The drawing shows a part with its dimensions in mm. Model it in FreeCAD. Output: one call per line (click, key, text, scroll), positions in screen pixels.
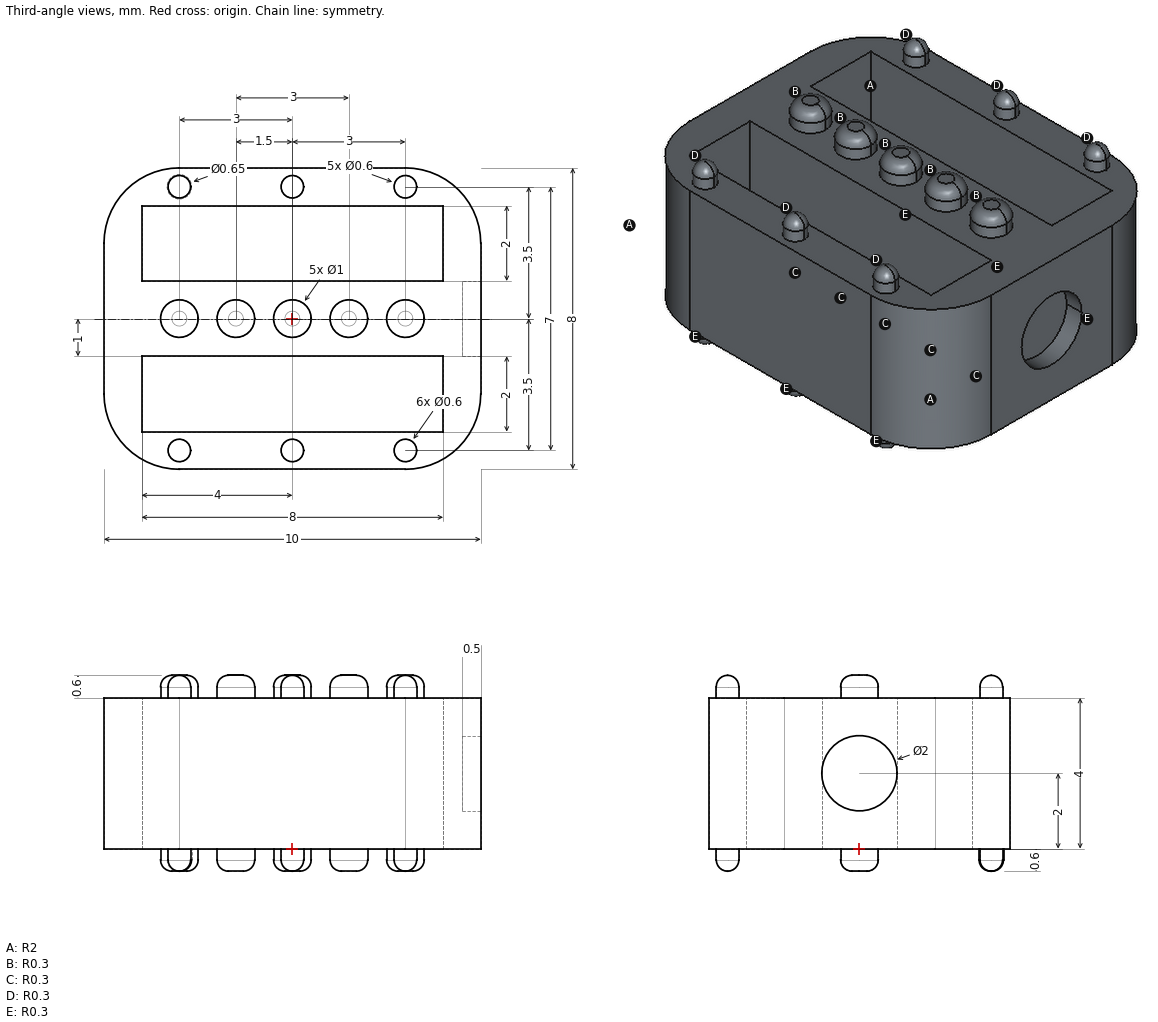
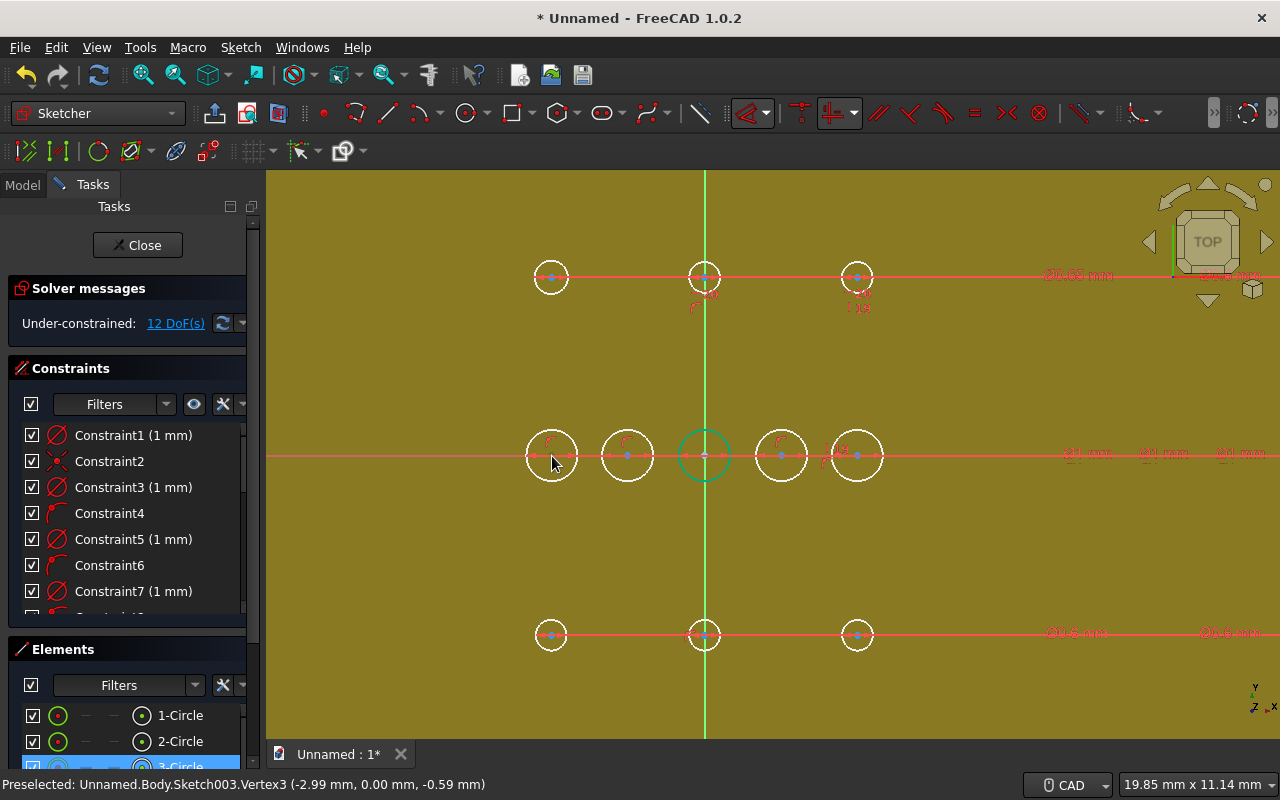
click(551, 277)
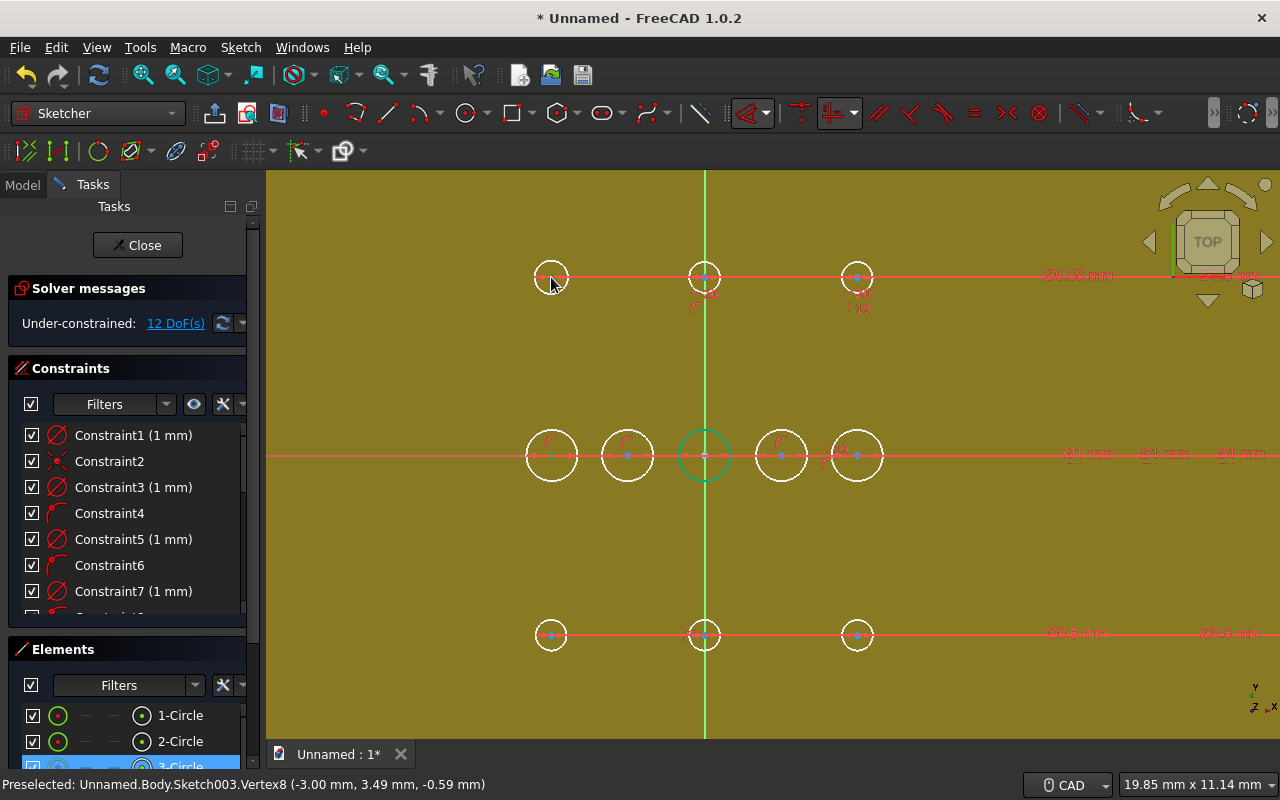
click(856, 114)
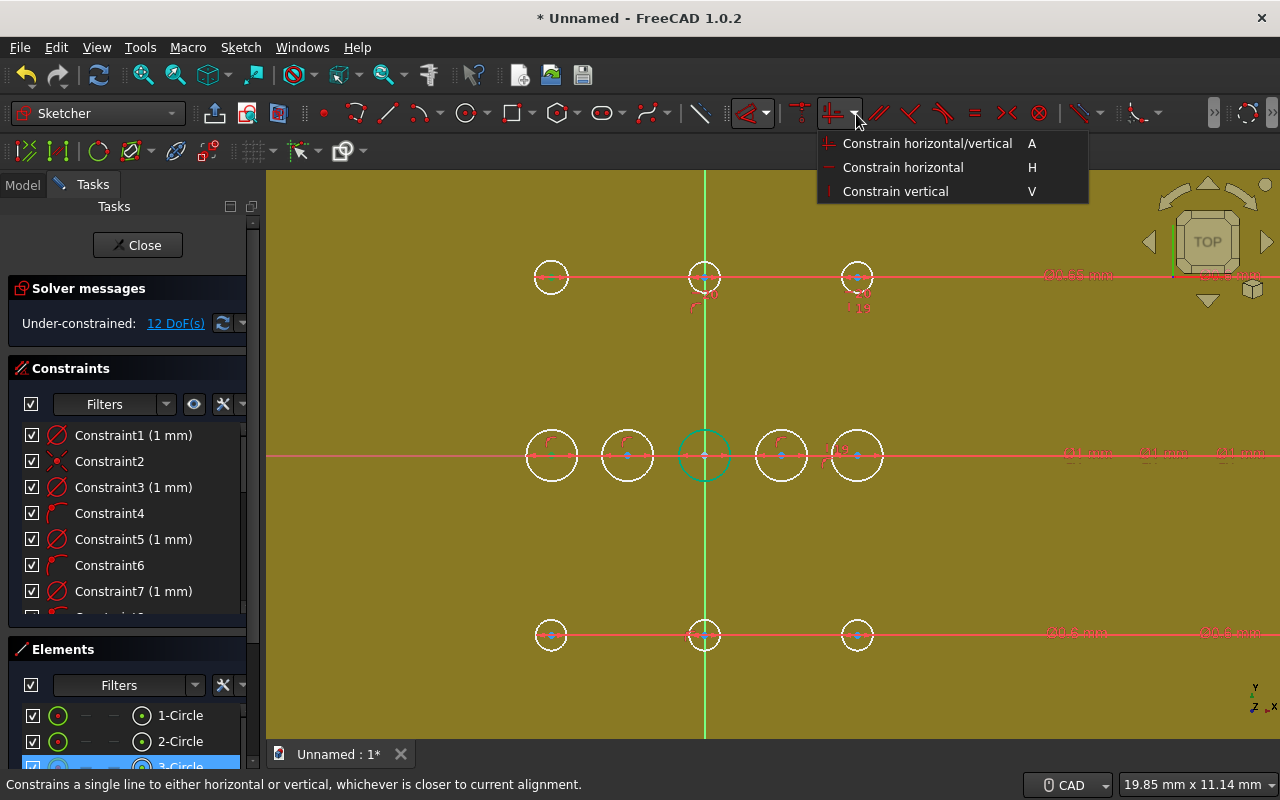
click(953, 191)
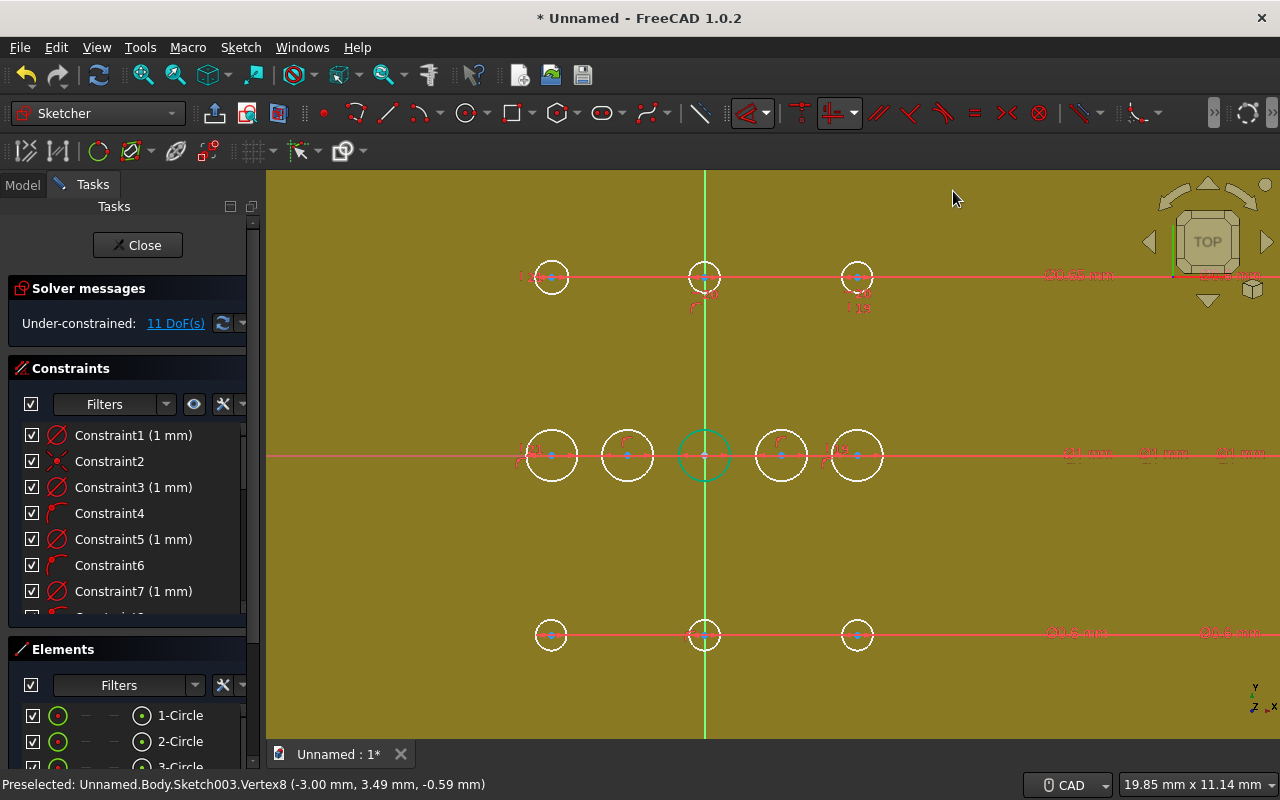
click(705, 277)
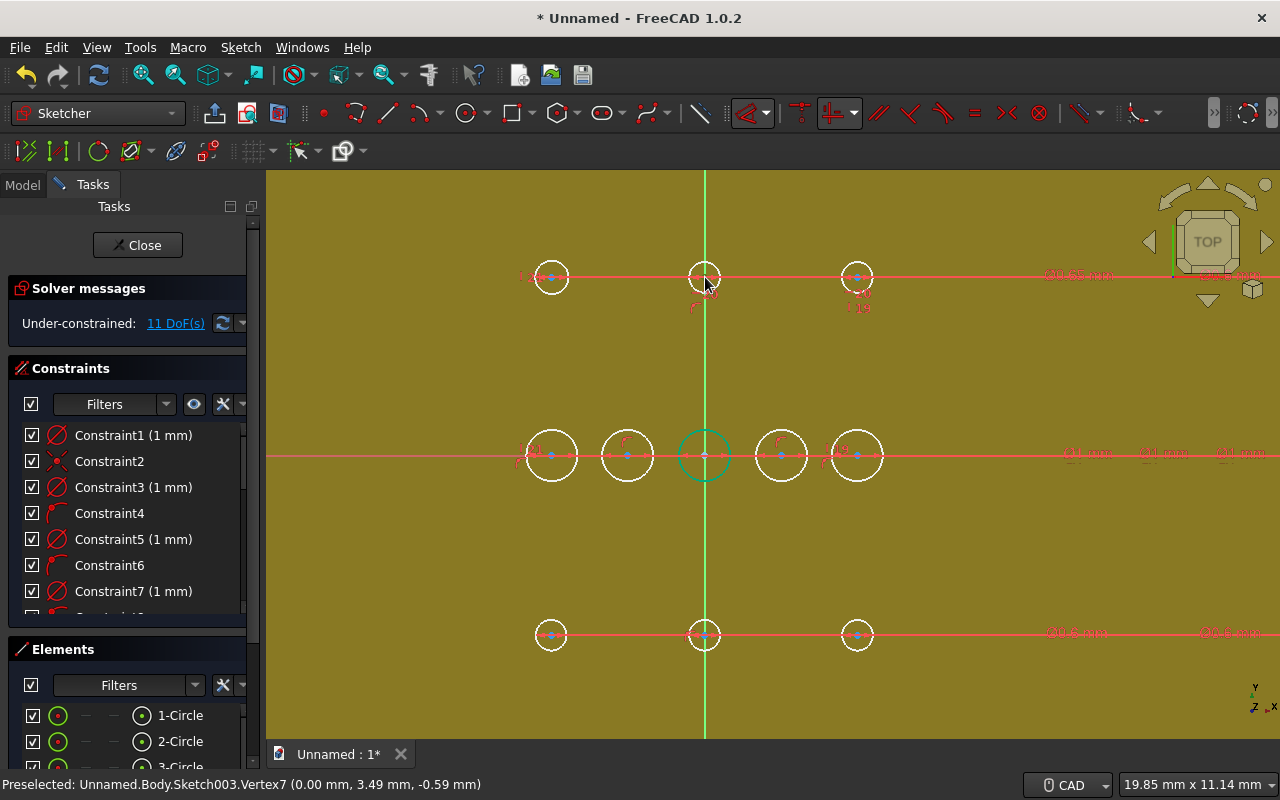
click(552, 277)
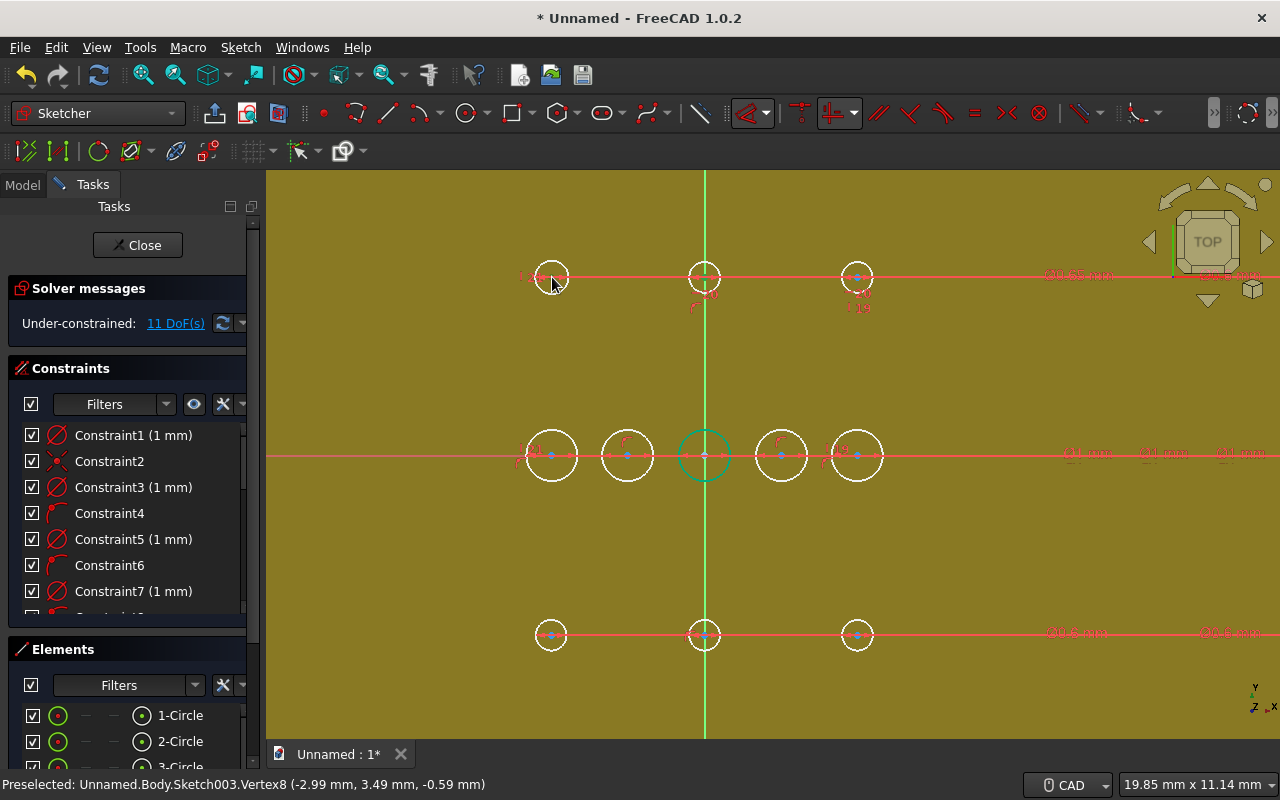
key(h)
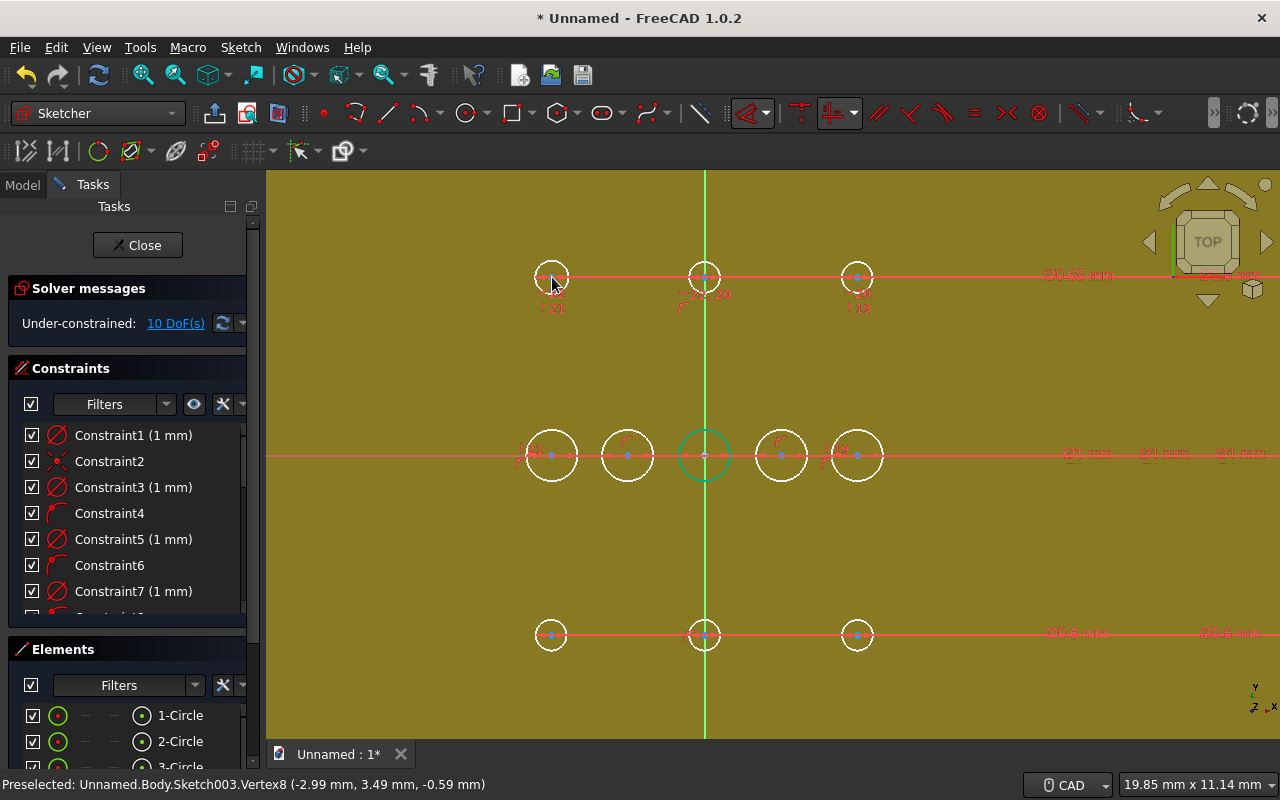
click(857, 456)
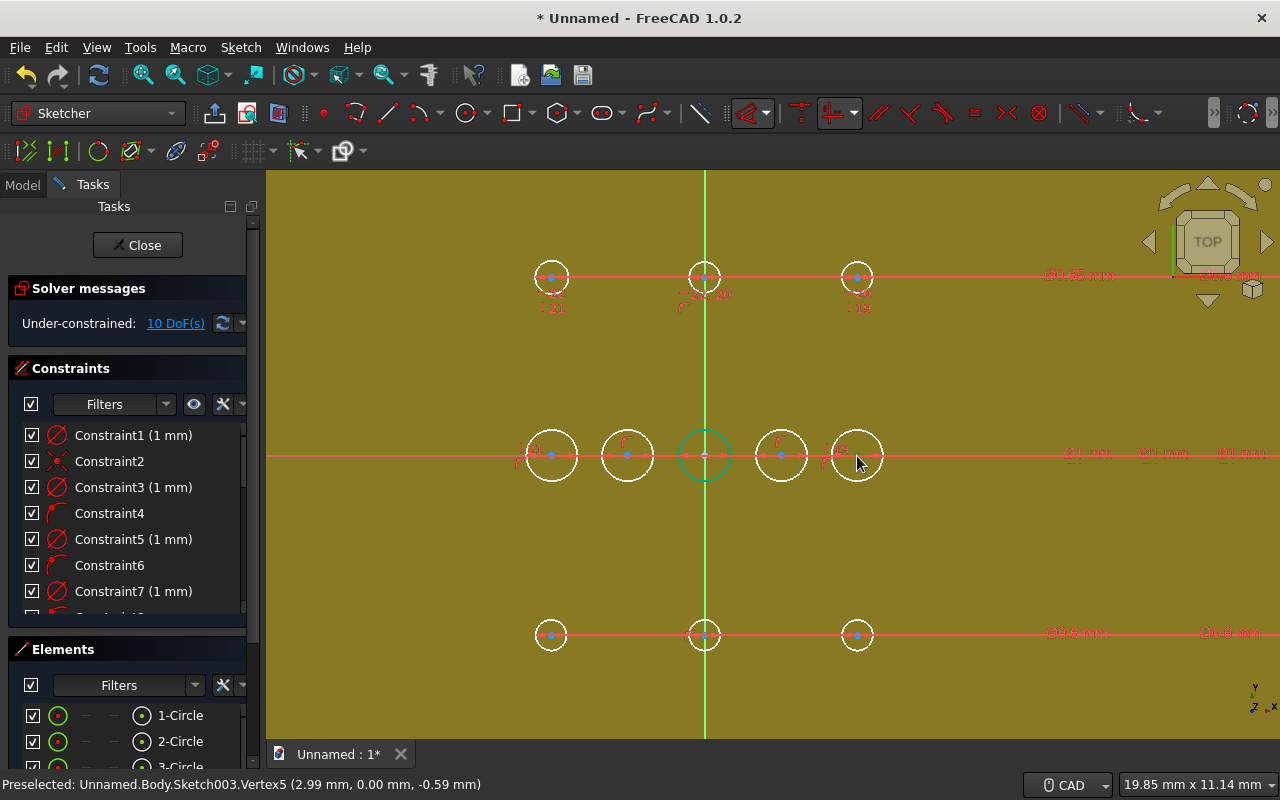
click(858, 635)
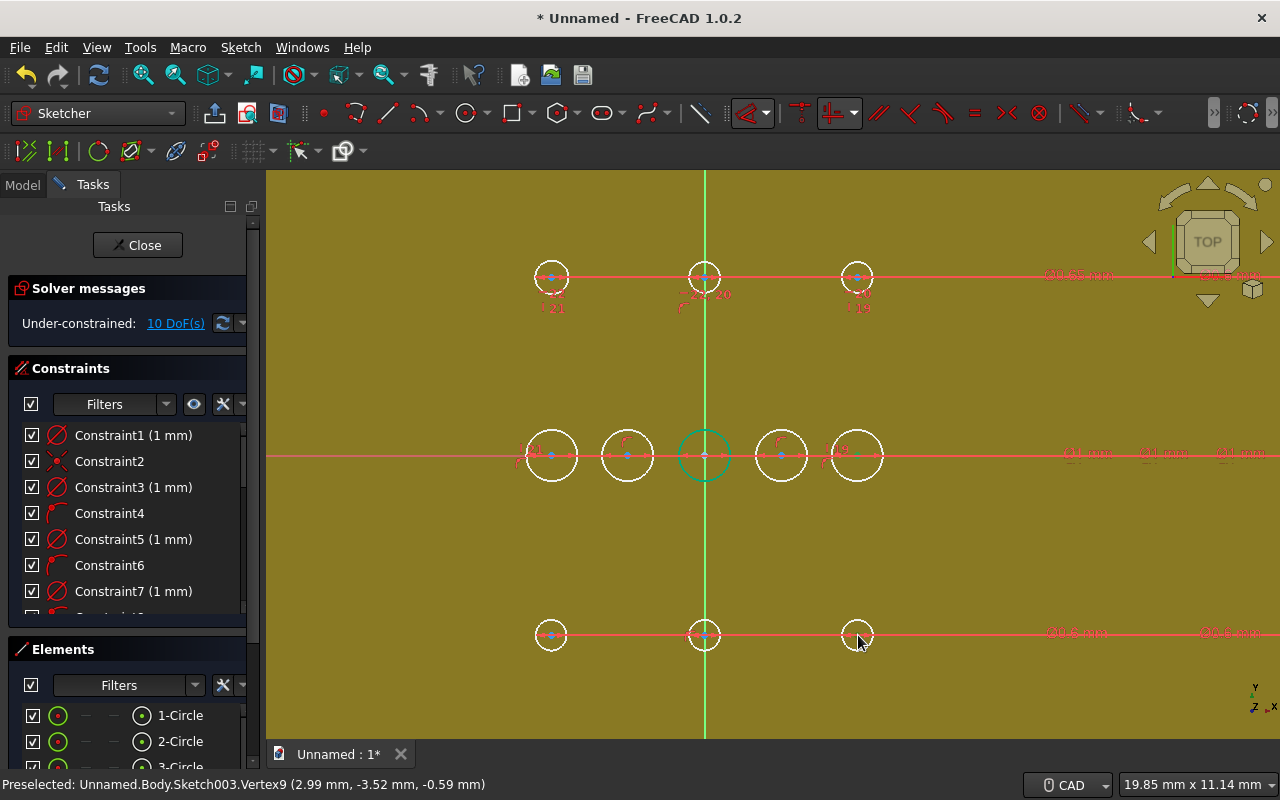
key(v)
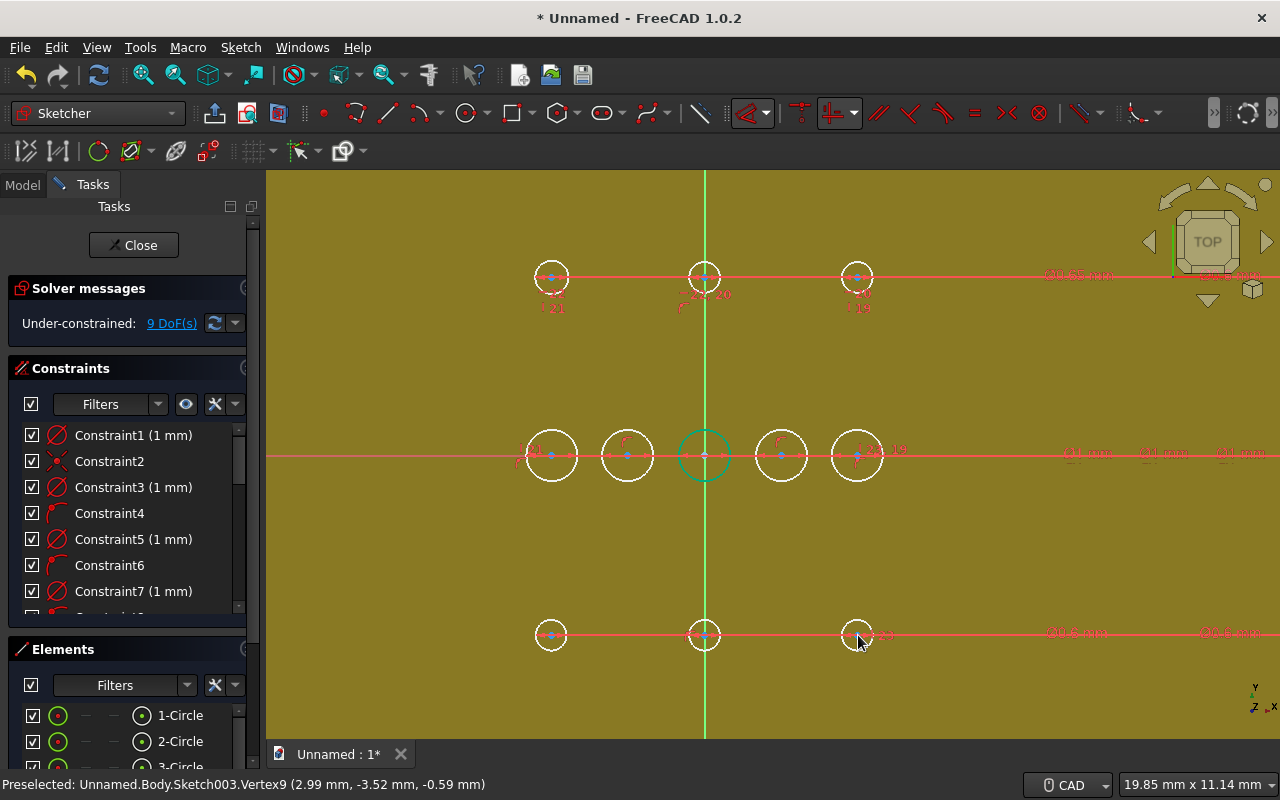
click(857, 635)